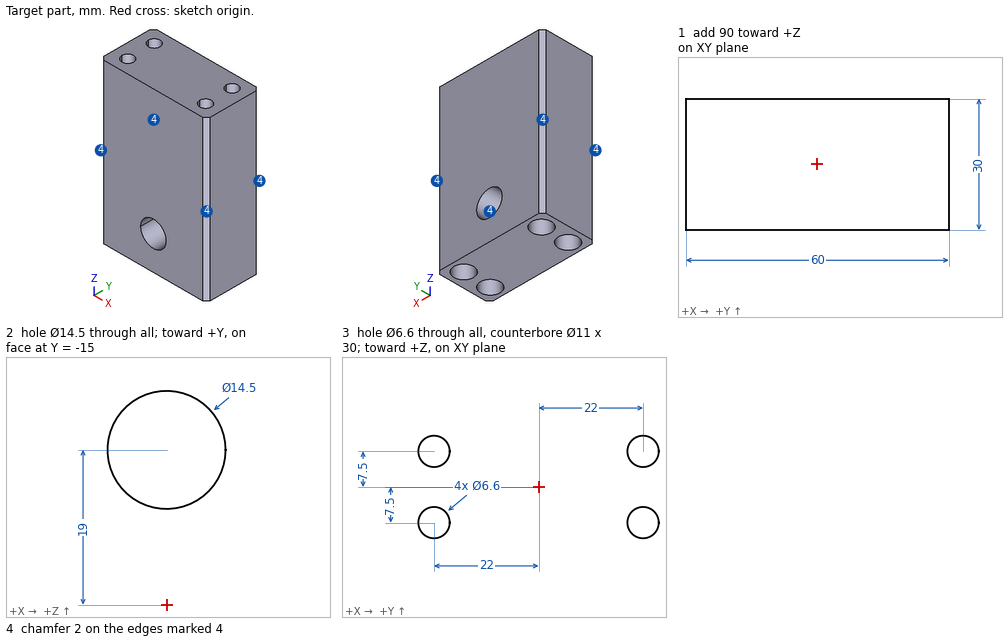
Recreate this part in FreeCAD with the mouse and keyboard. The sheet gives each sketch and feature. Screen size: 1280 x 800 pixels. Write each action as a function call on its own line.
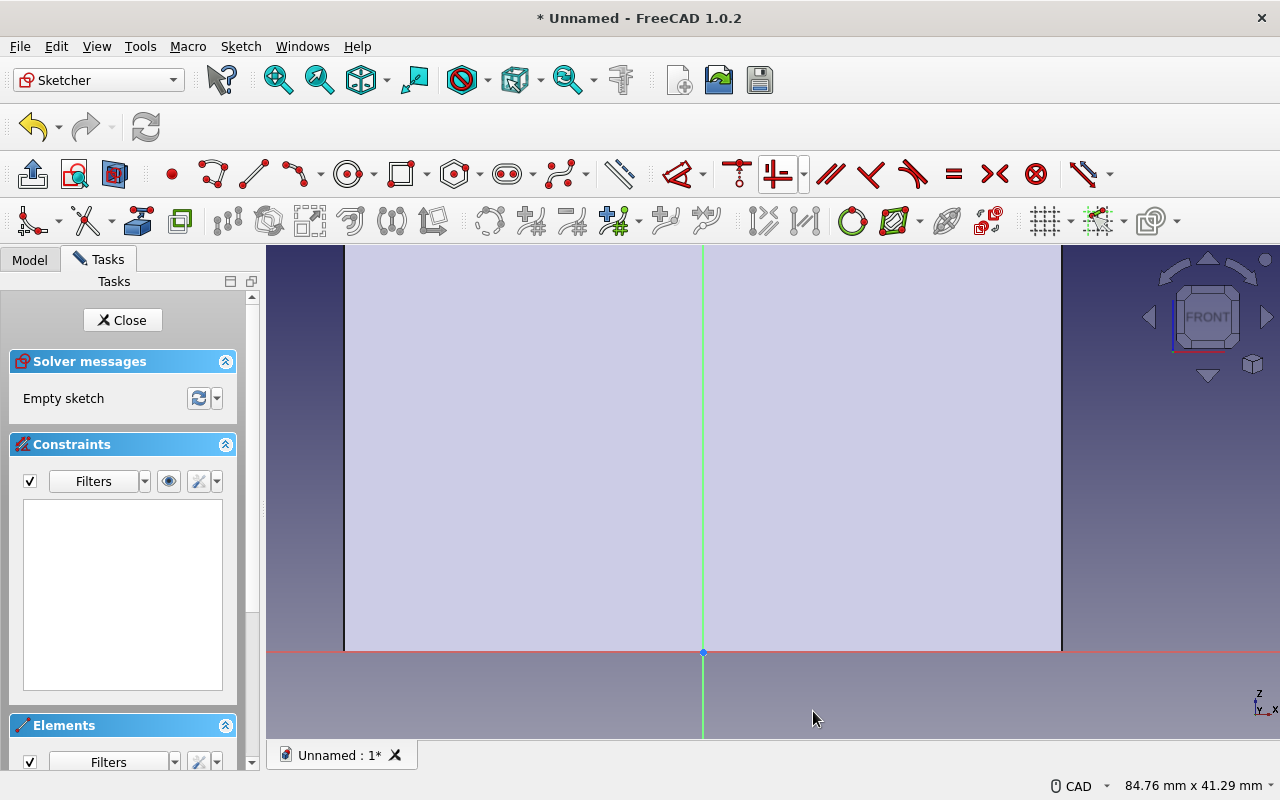
key(g)
key(c)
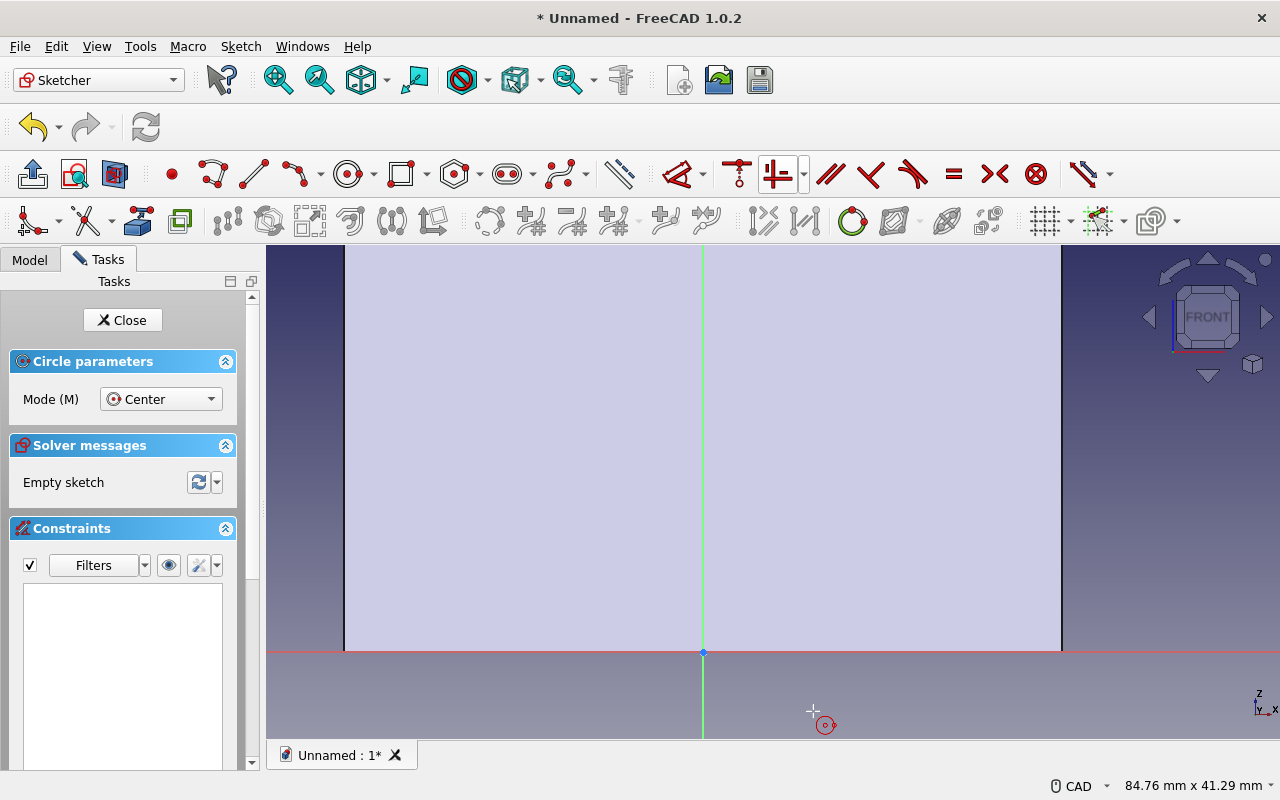
click(703, 425)
click(765, 364)
key(Escape)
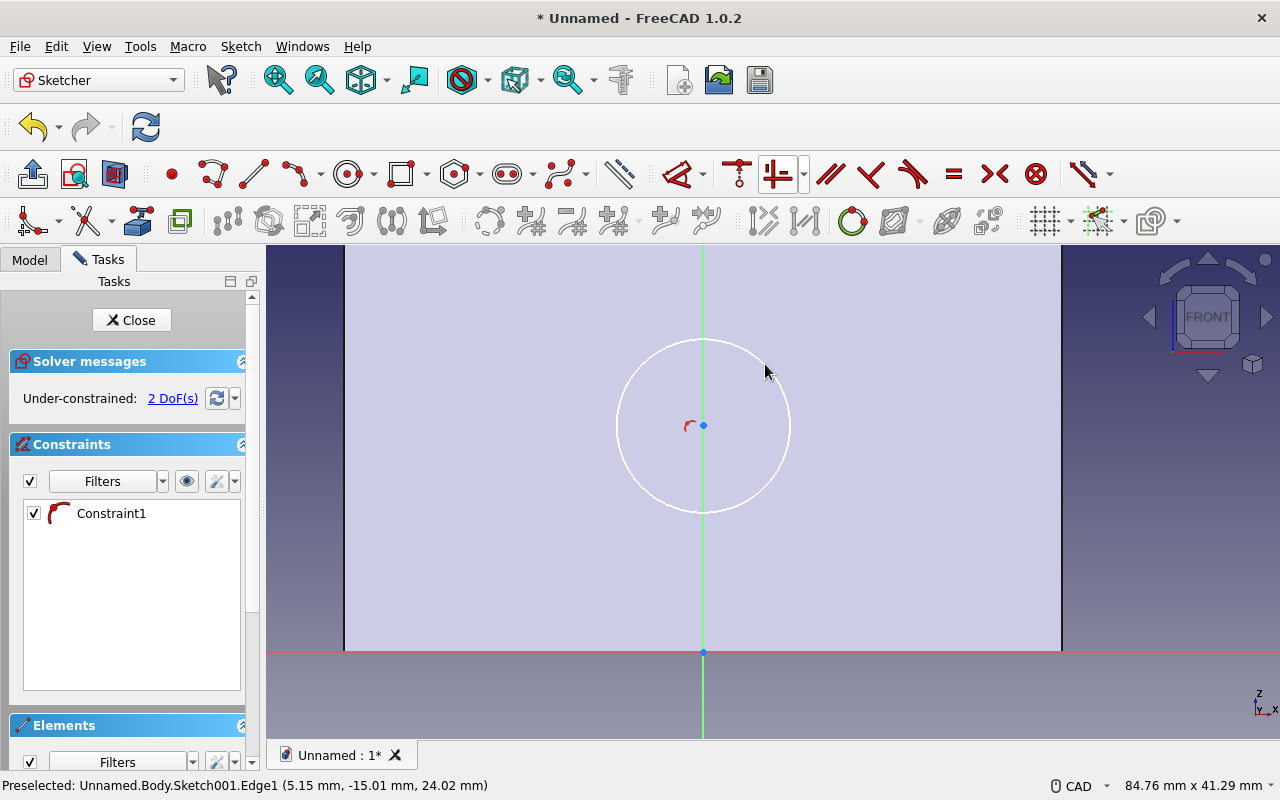
click(676, 174)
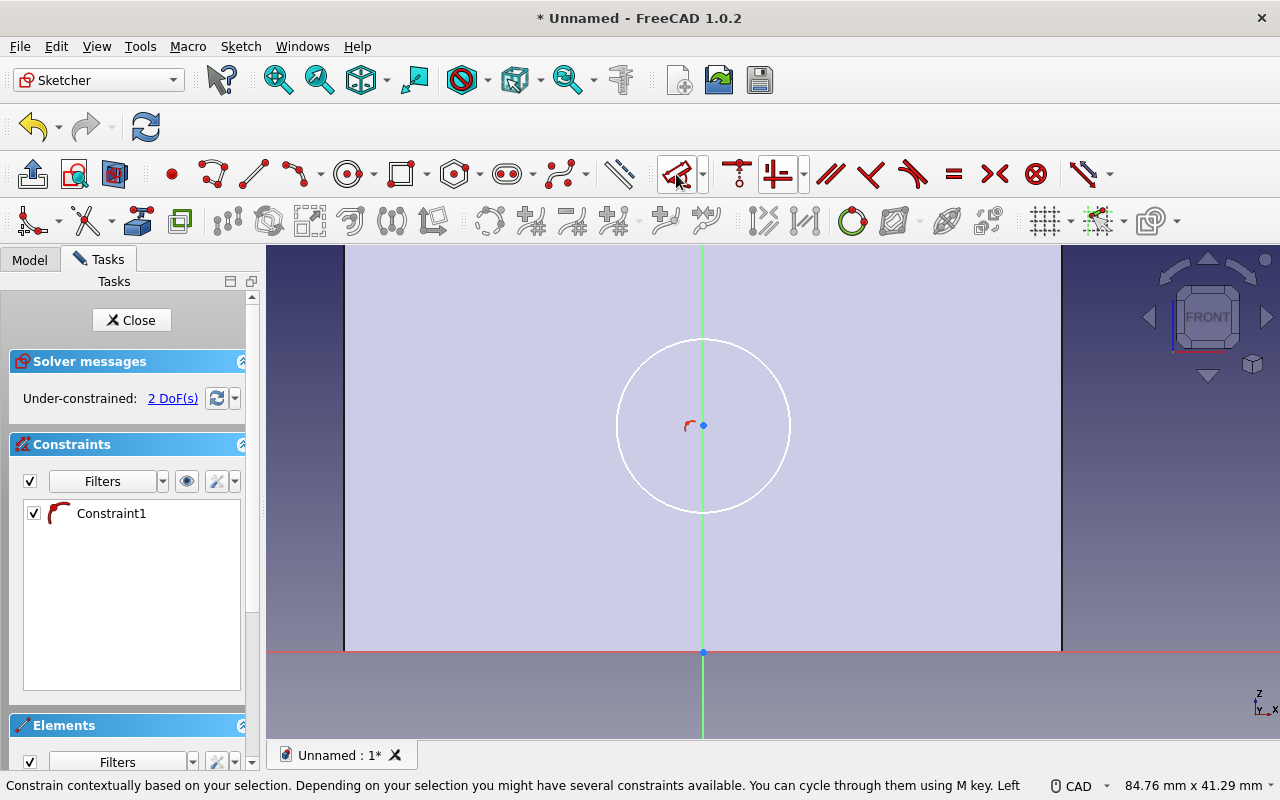
click(764, 364)
click(786, 341)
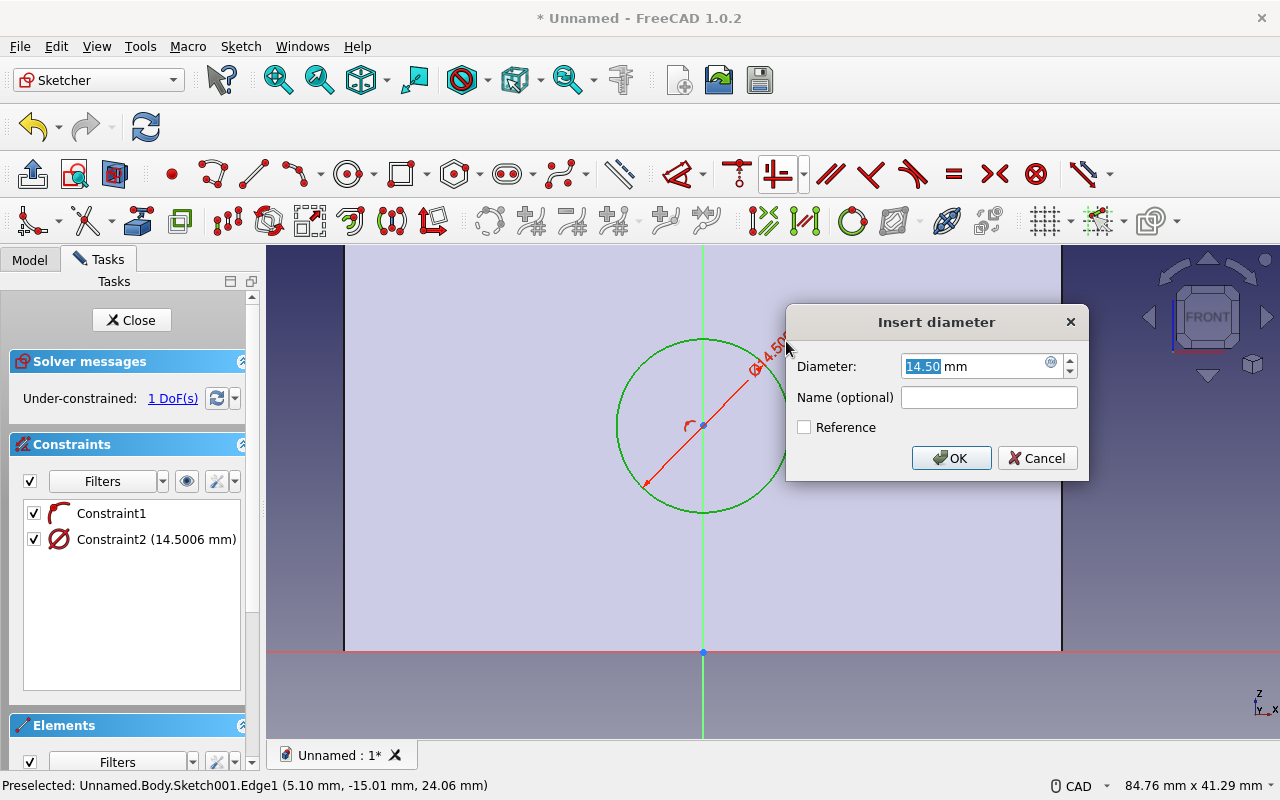
text(14.5)
key(Return)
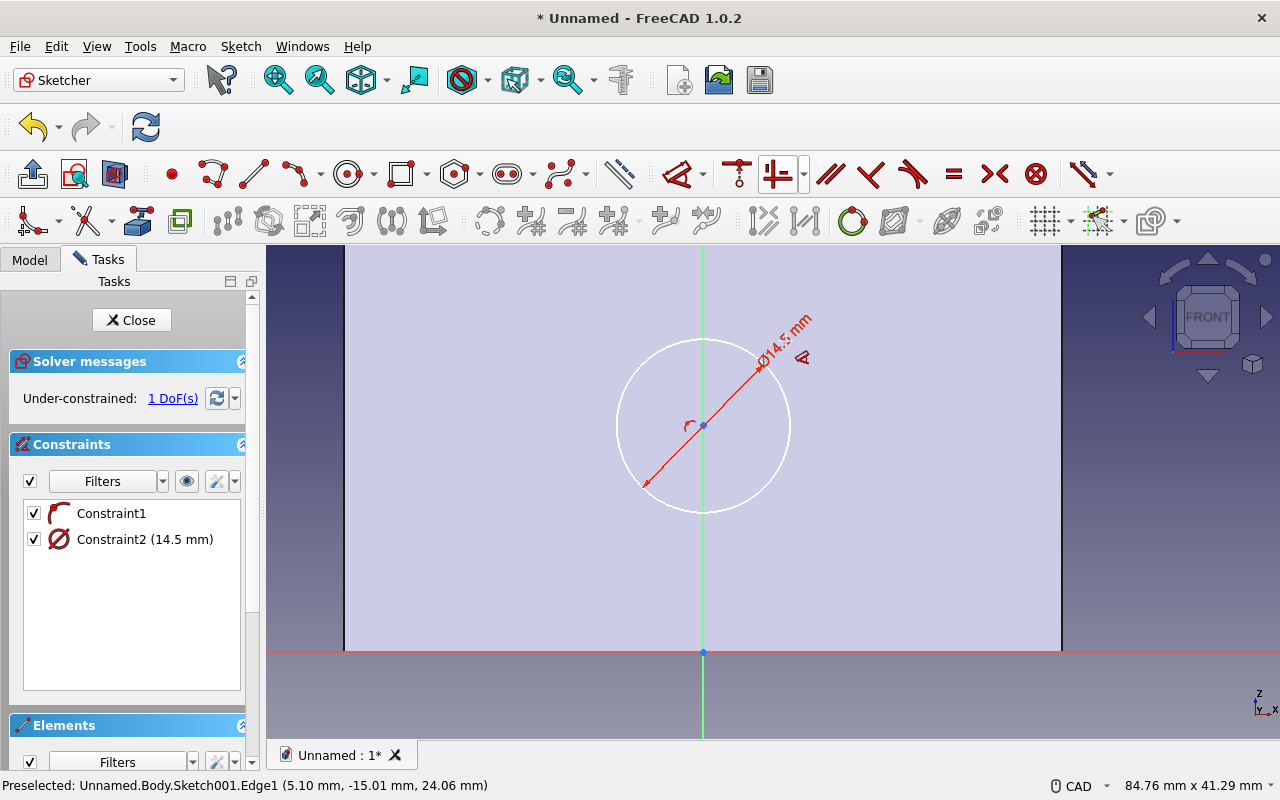
click(703, 426)
click(737, 539)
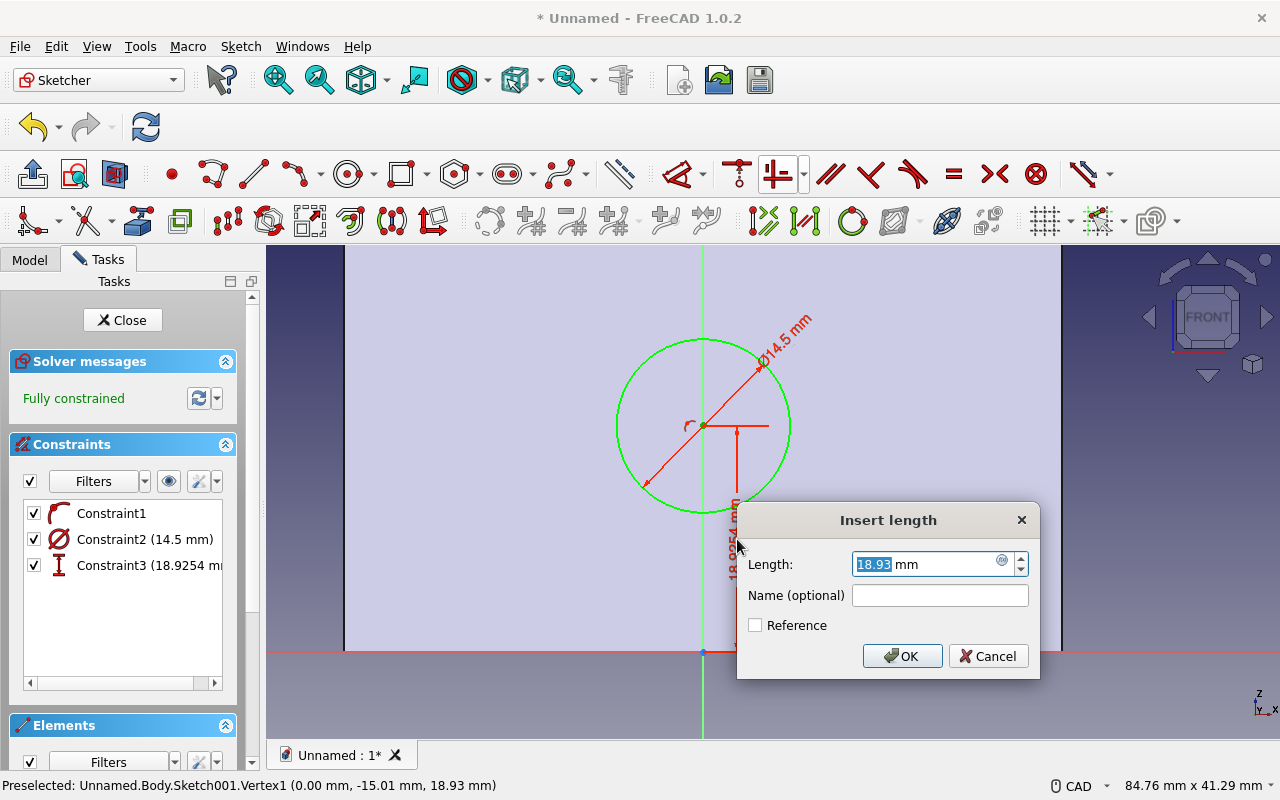
text(19)
key(Return)
key(Escape)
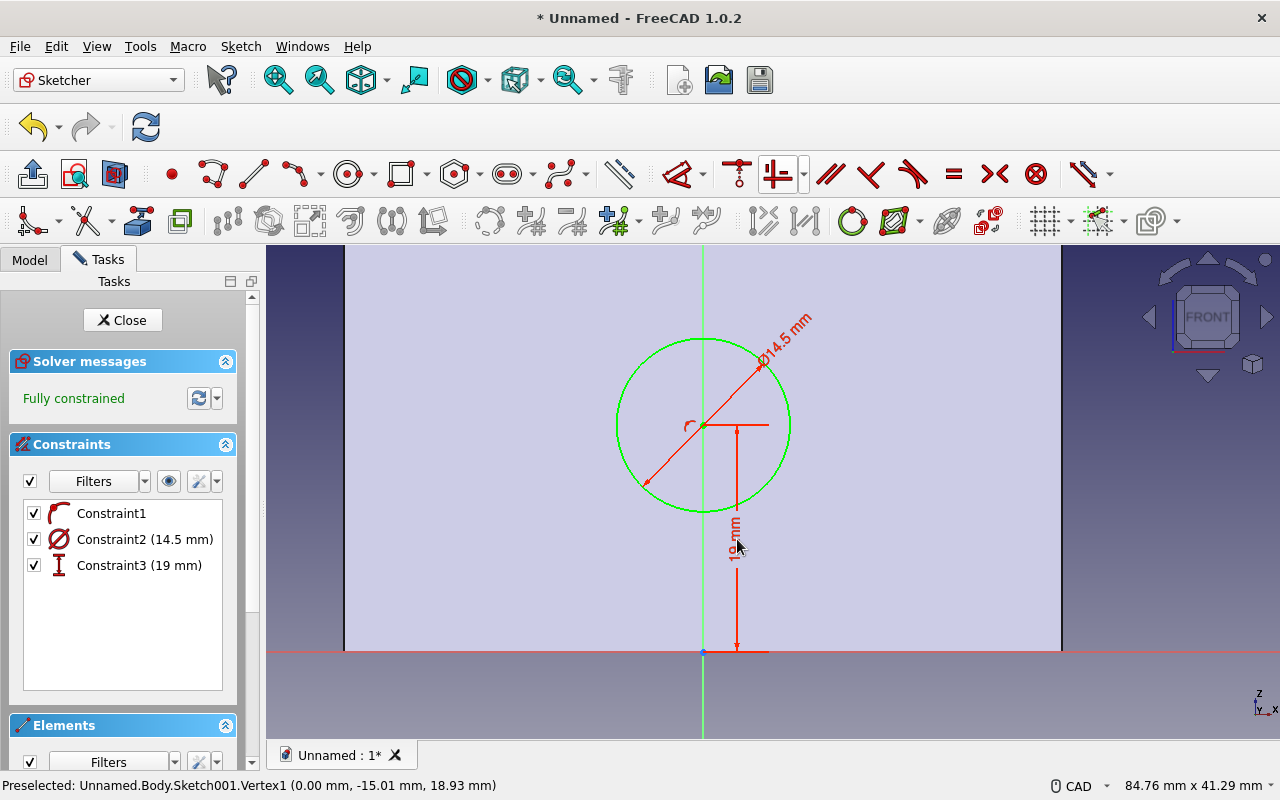
click(123, 320)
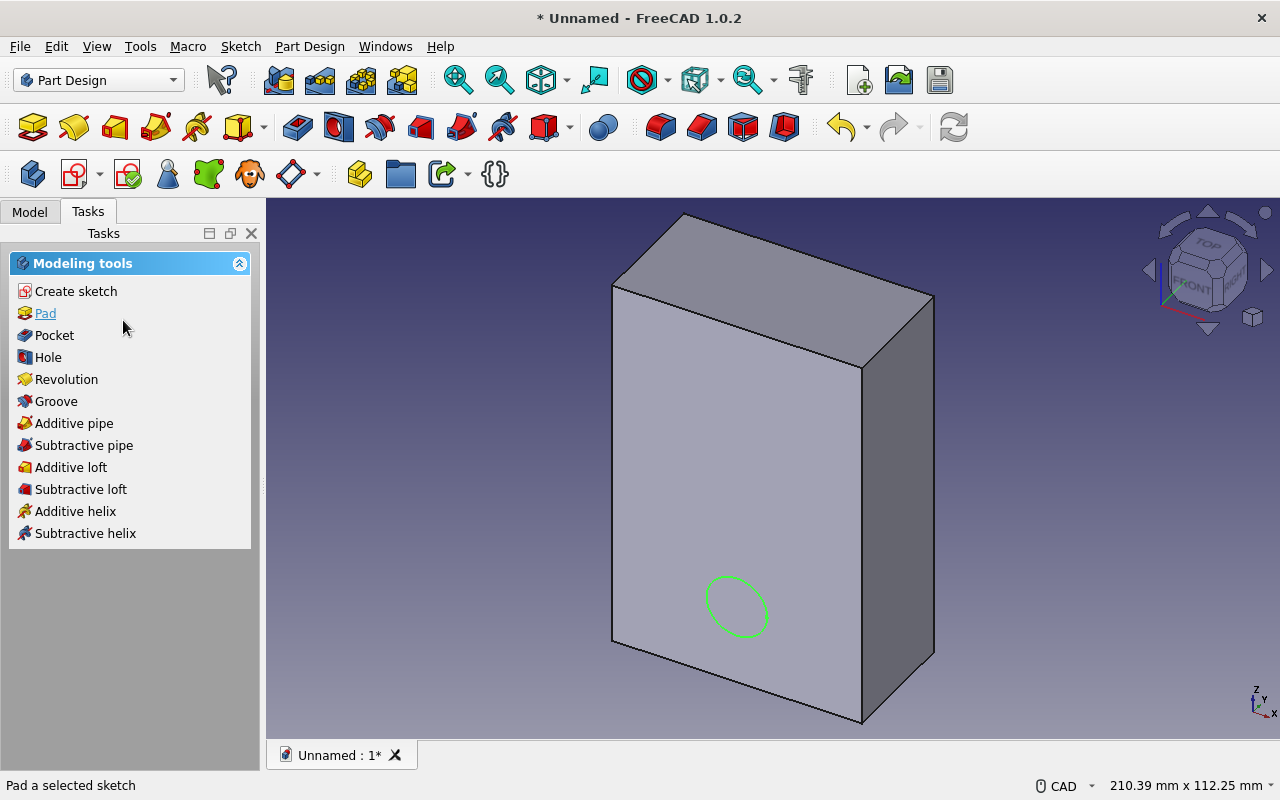
click(339, 128)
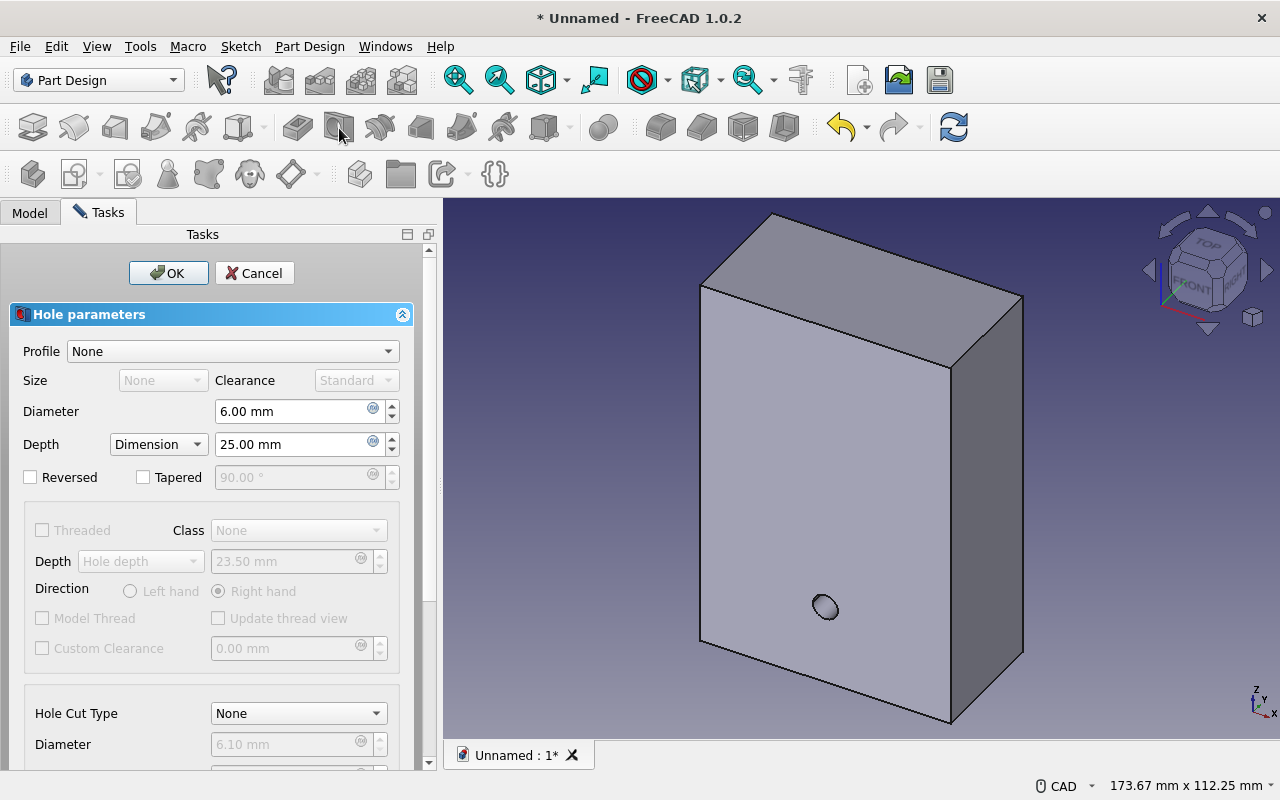
triple_click(300, 412)